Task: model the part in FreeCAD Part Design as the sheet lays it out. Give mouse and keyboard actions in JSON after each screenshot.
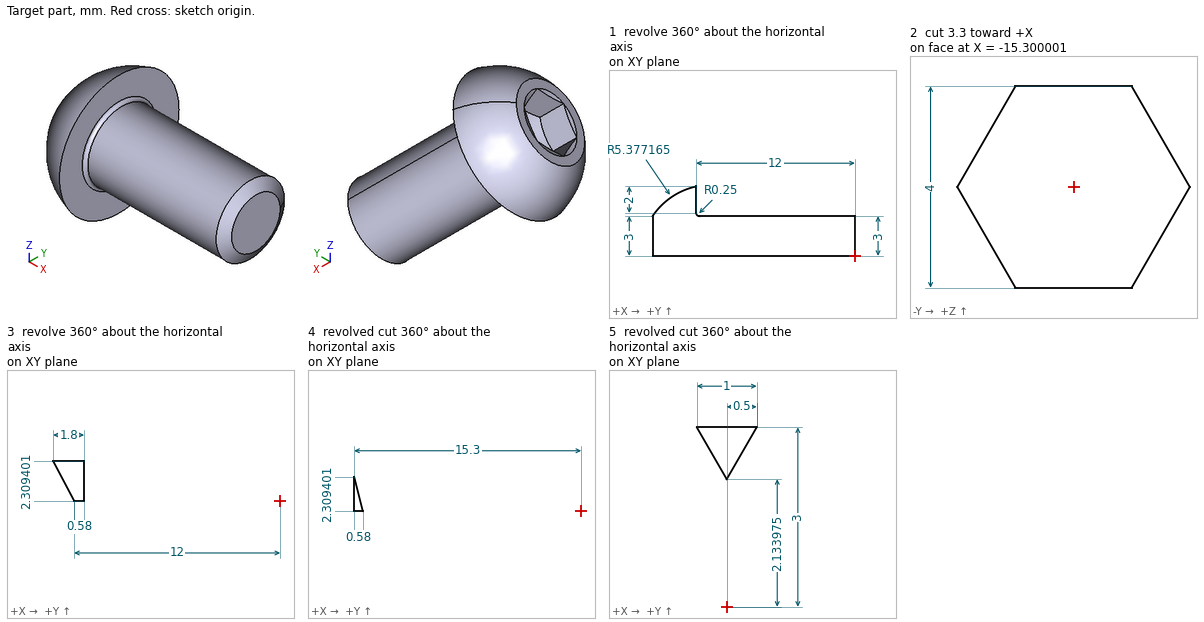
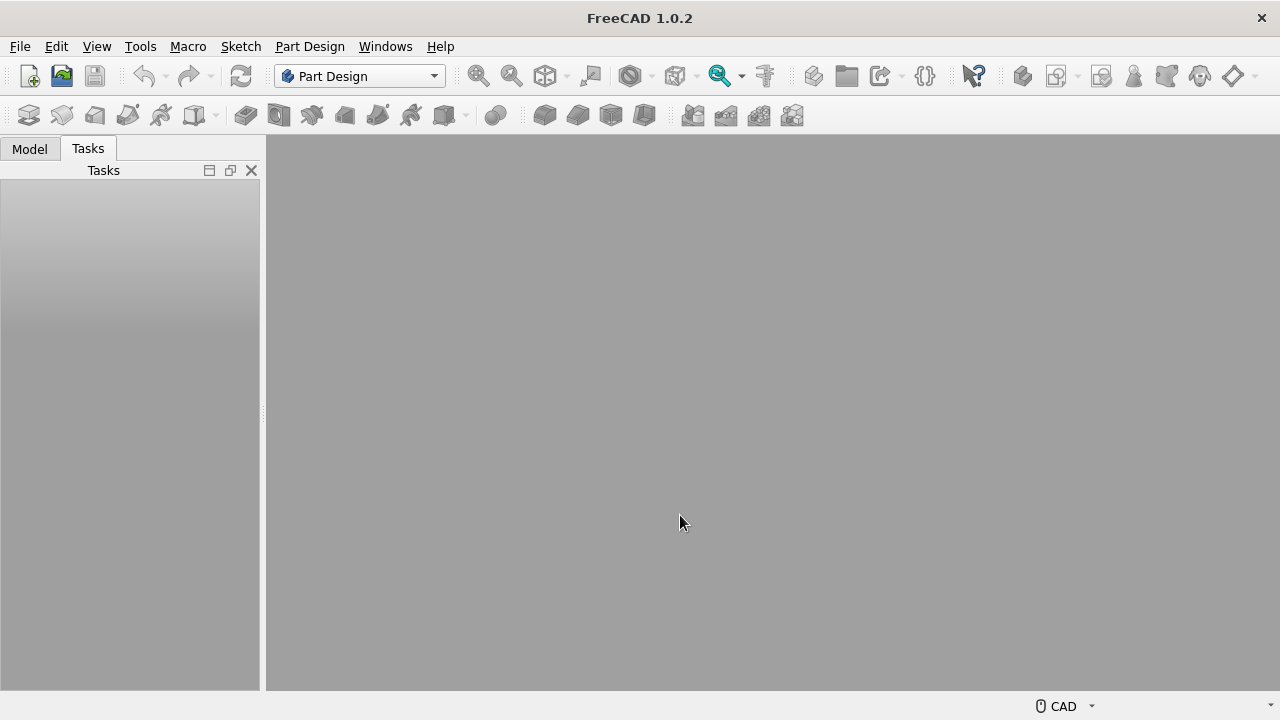
{"action": "left_click", "coordinate": [29, 76]}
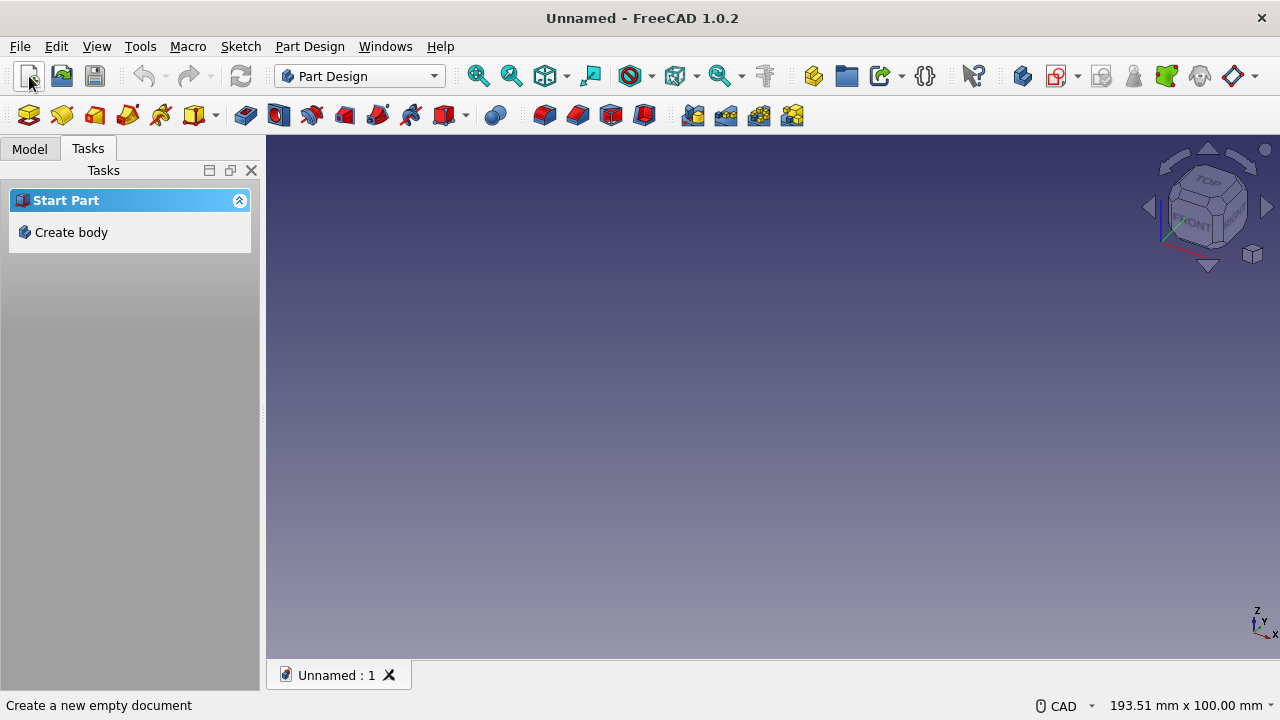
{"action": "left_click", "coordinate": [1056, 76]}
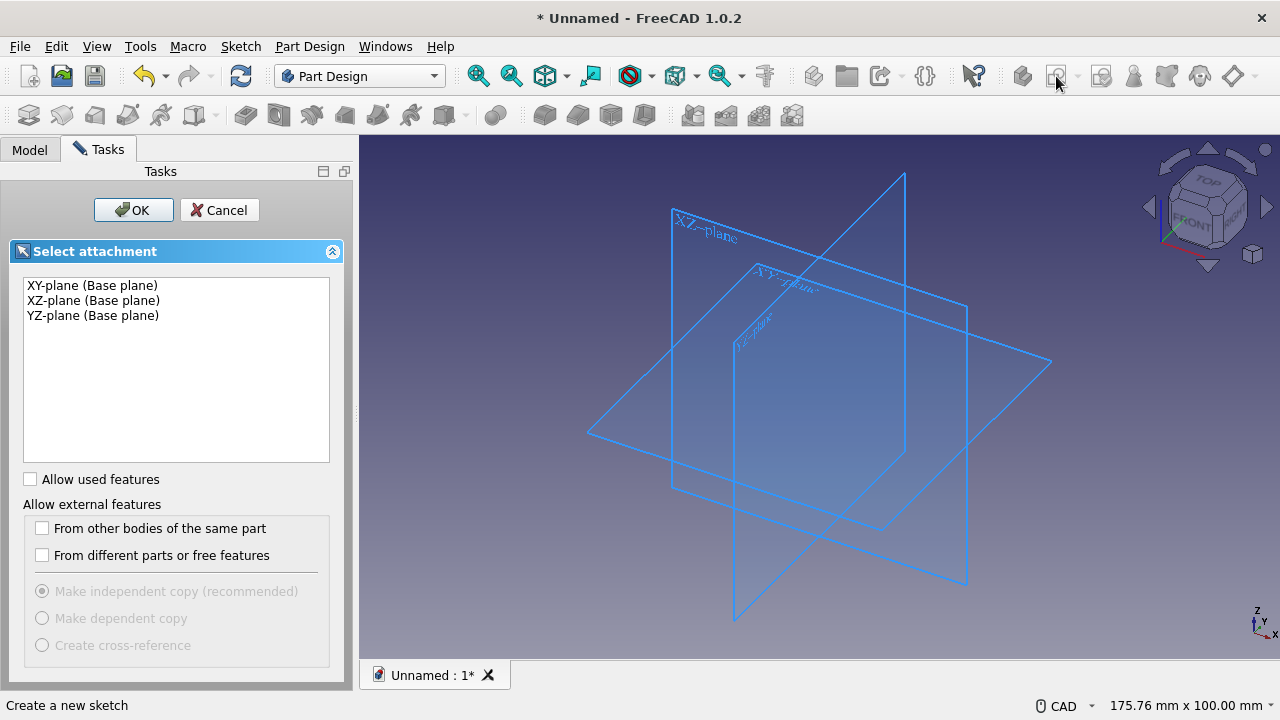
{"action": "left_click", "coordinate": [84, 286]}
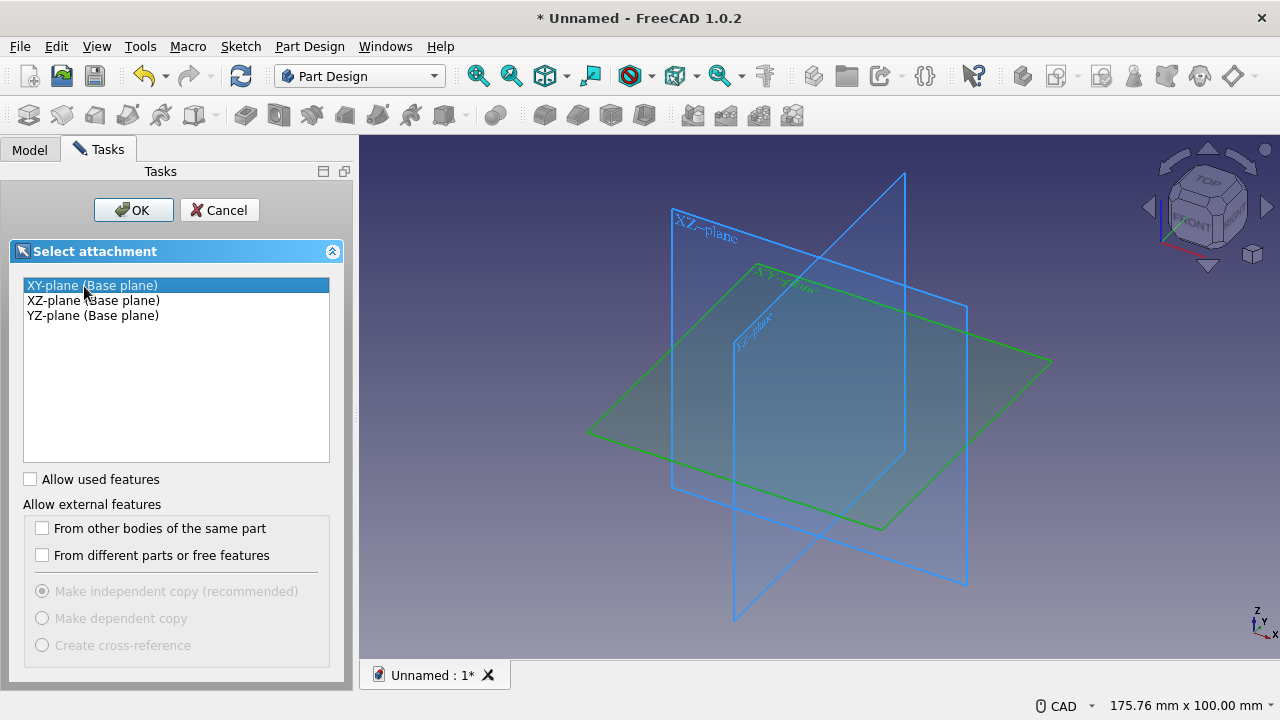
{"action": "left_click", "coordinate": [134, 210]}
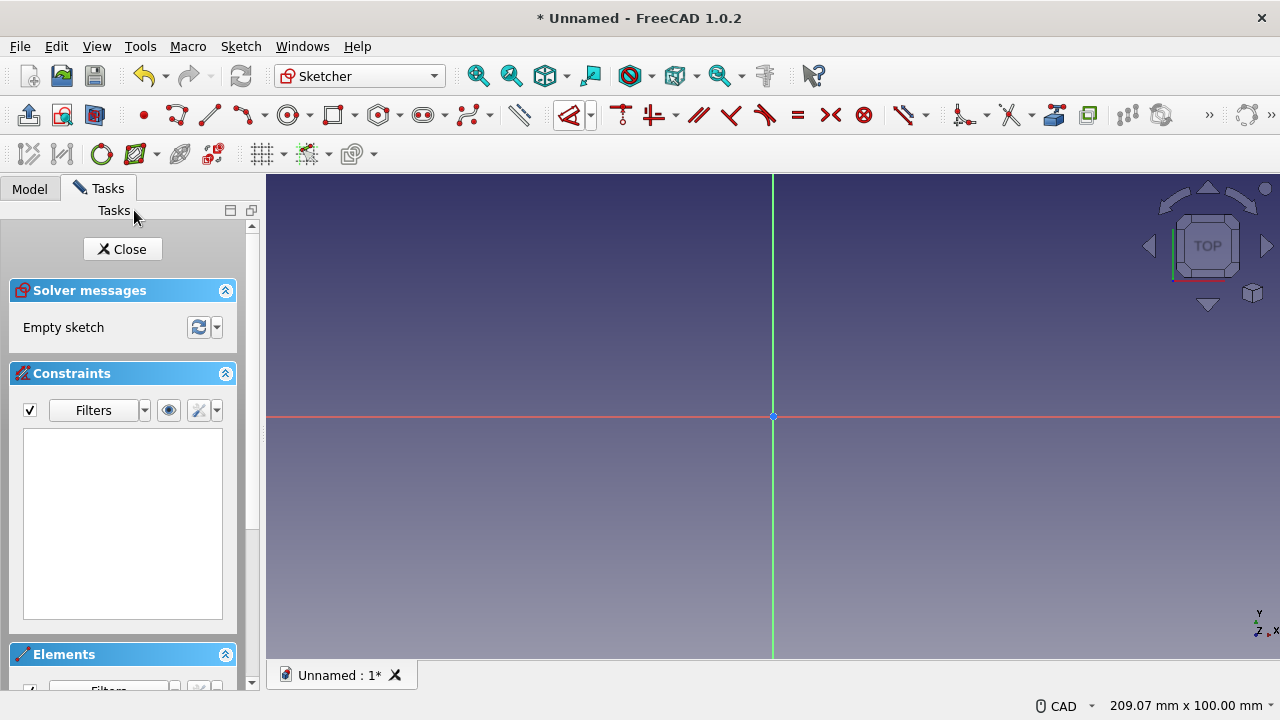
{"action": "scroll", "coordinate": [741, 402], "scroll_direction": "up", "scroll_amount": 10}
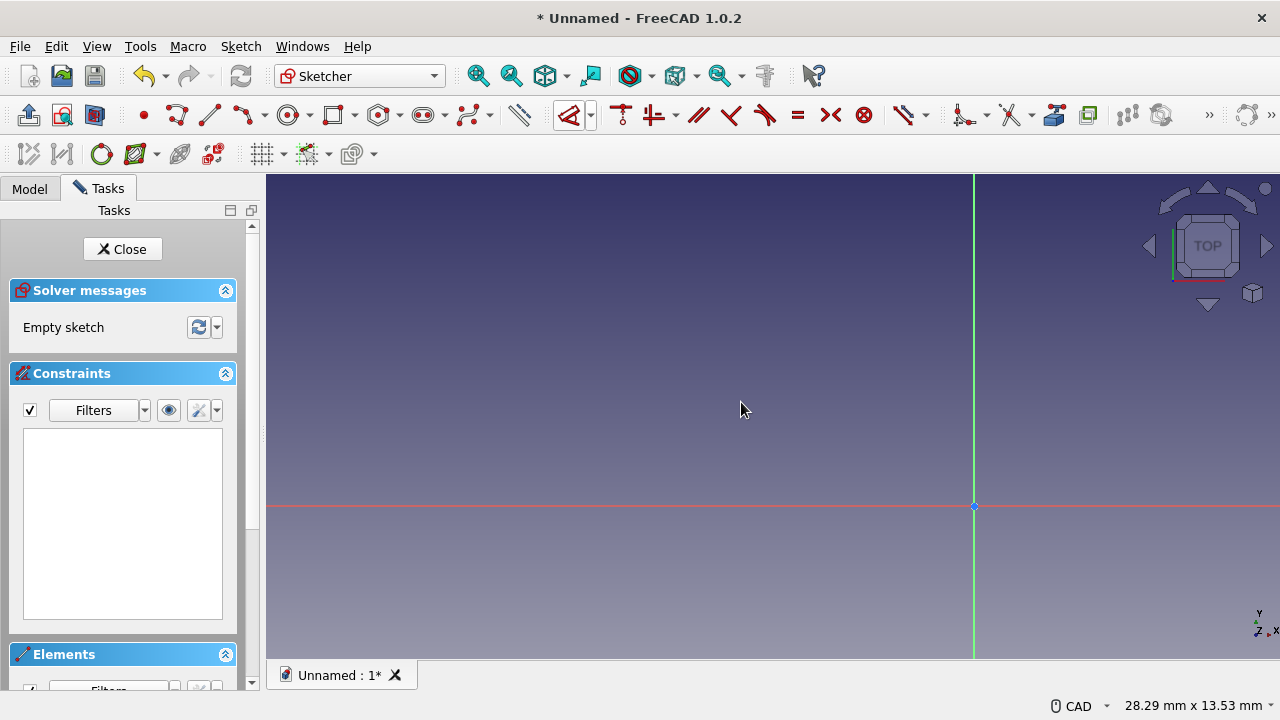
{"action": "key", "text": "g l"}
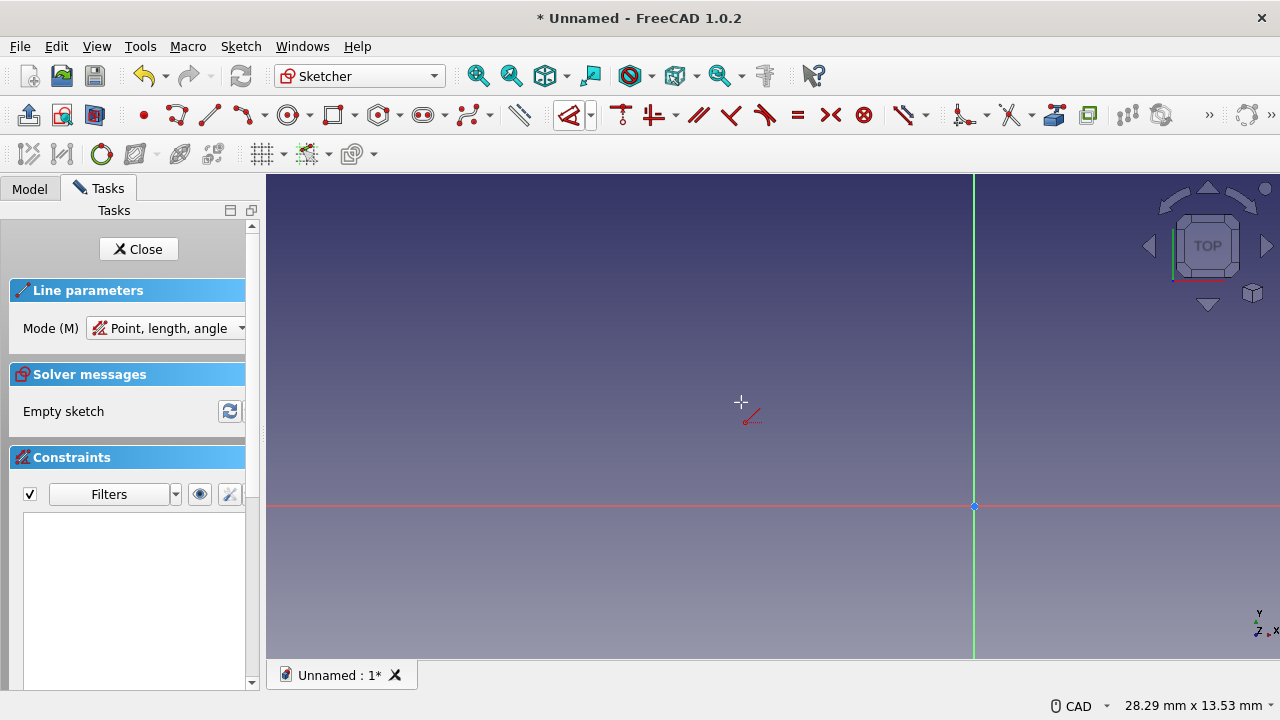
{"action": "left_click", "coordinate": [544, 390]}
{"action": "left_click", "coordinate": [544, 318]}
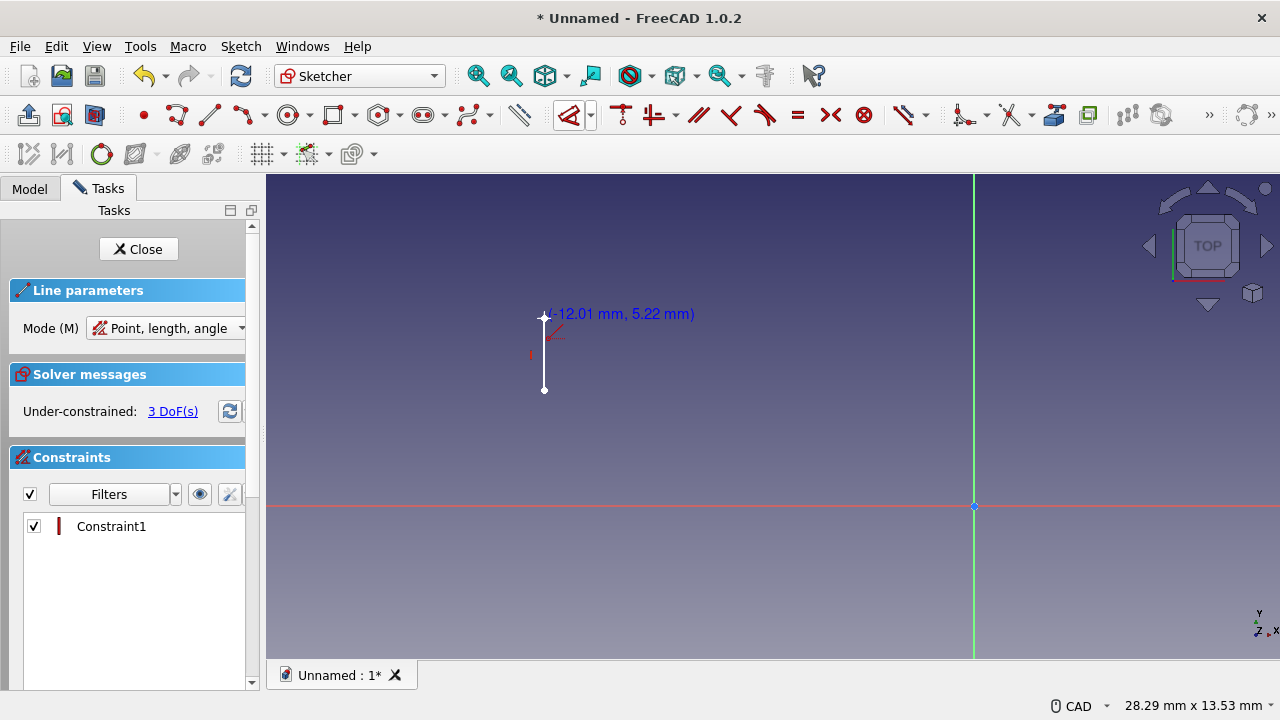
{"action": "left_click", "coordinate": [177, 116]}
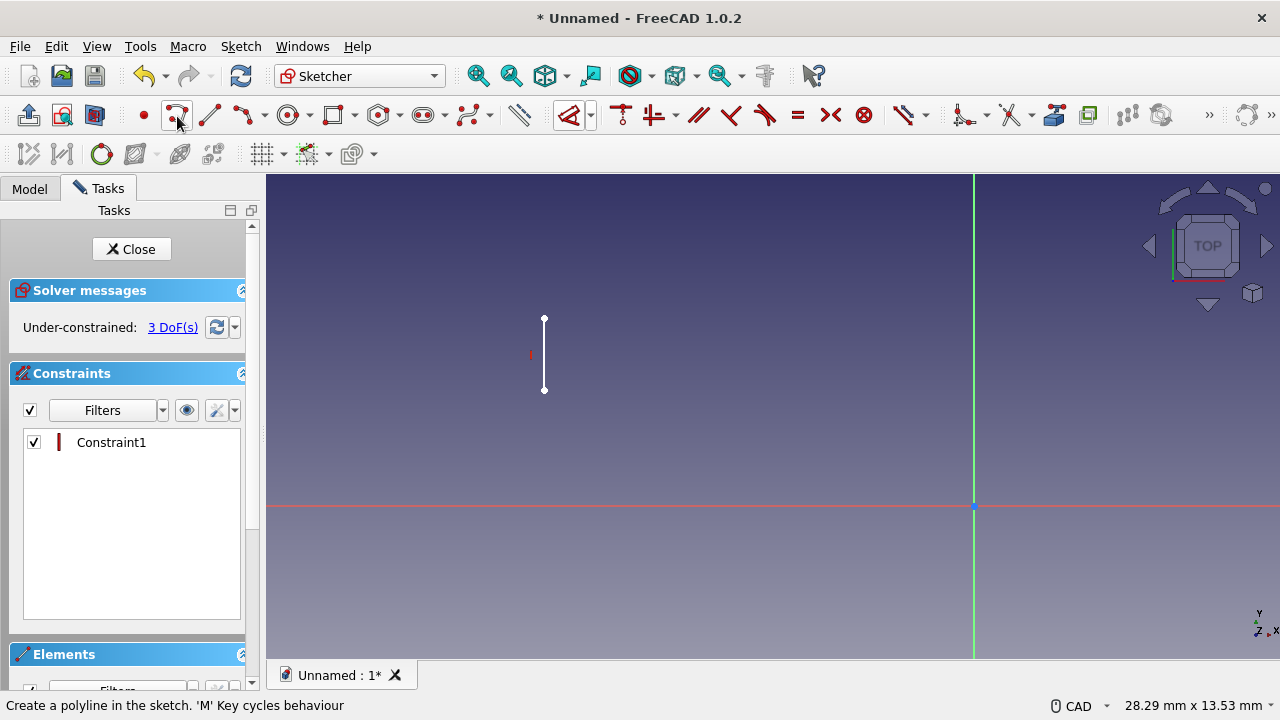
{"action": "left_click", "coordinate": [426, 399]}
{"action": "left_click", "coordinate": [426, 506]}
{"action": "left_click", "coordinate": [974, 506]}
{"action": "left_click", "coordinate": [965, 399]}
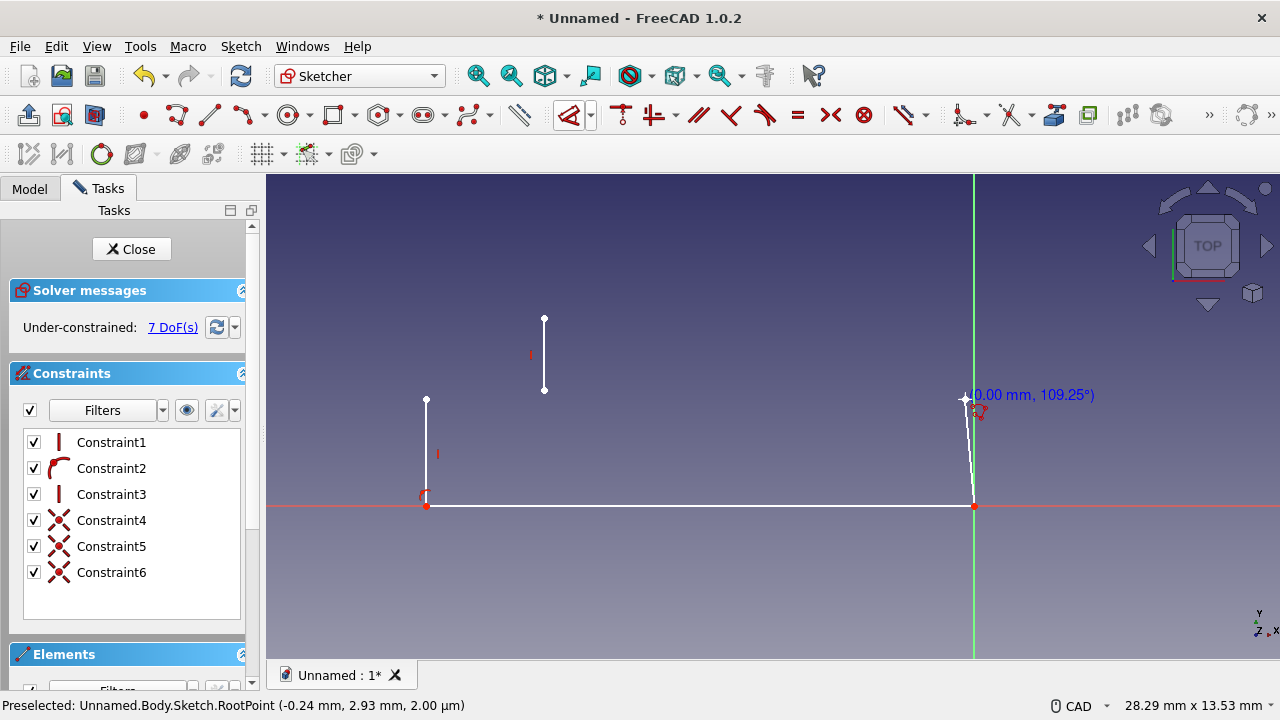
{"action": "scroll", "coordinate": [553, 399], "scroll_direction": "up", "scroll_amount": 2}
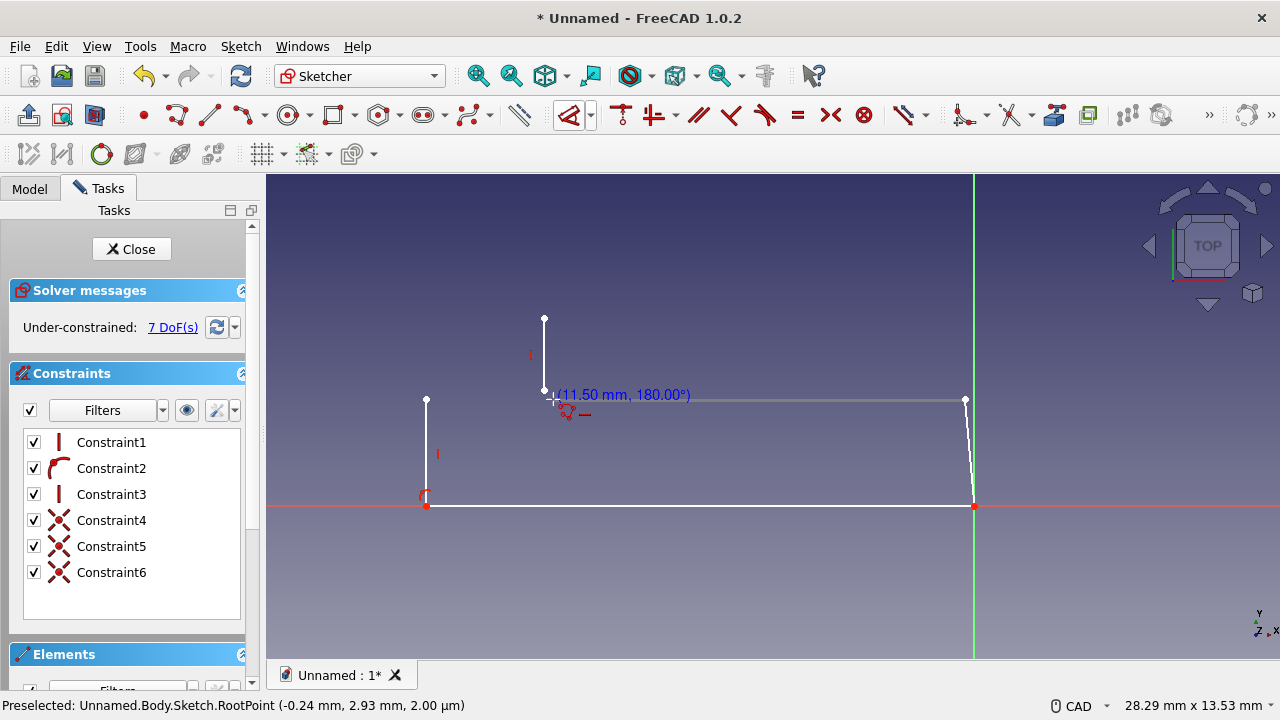
{"action": "left_click", "coordinate": [553, 399]}
{"action": "right_click", "coordinate": [553, 399]}